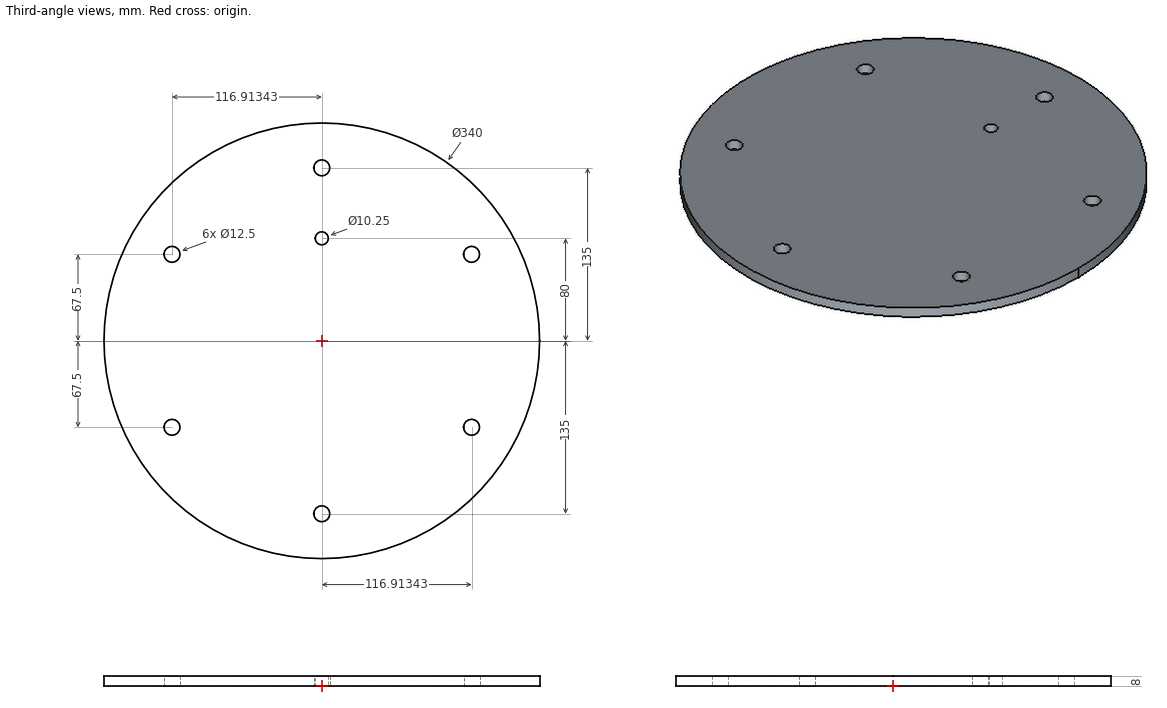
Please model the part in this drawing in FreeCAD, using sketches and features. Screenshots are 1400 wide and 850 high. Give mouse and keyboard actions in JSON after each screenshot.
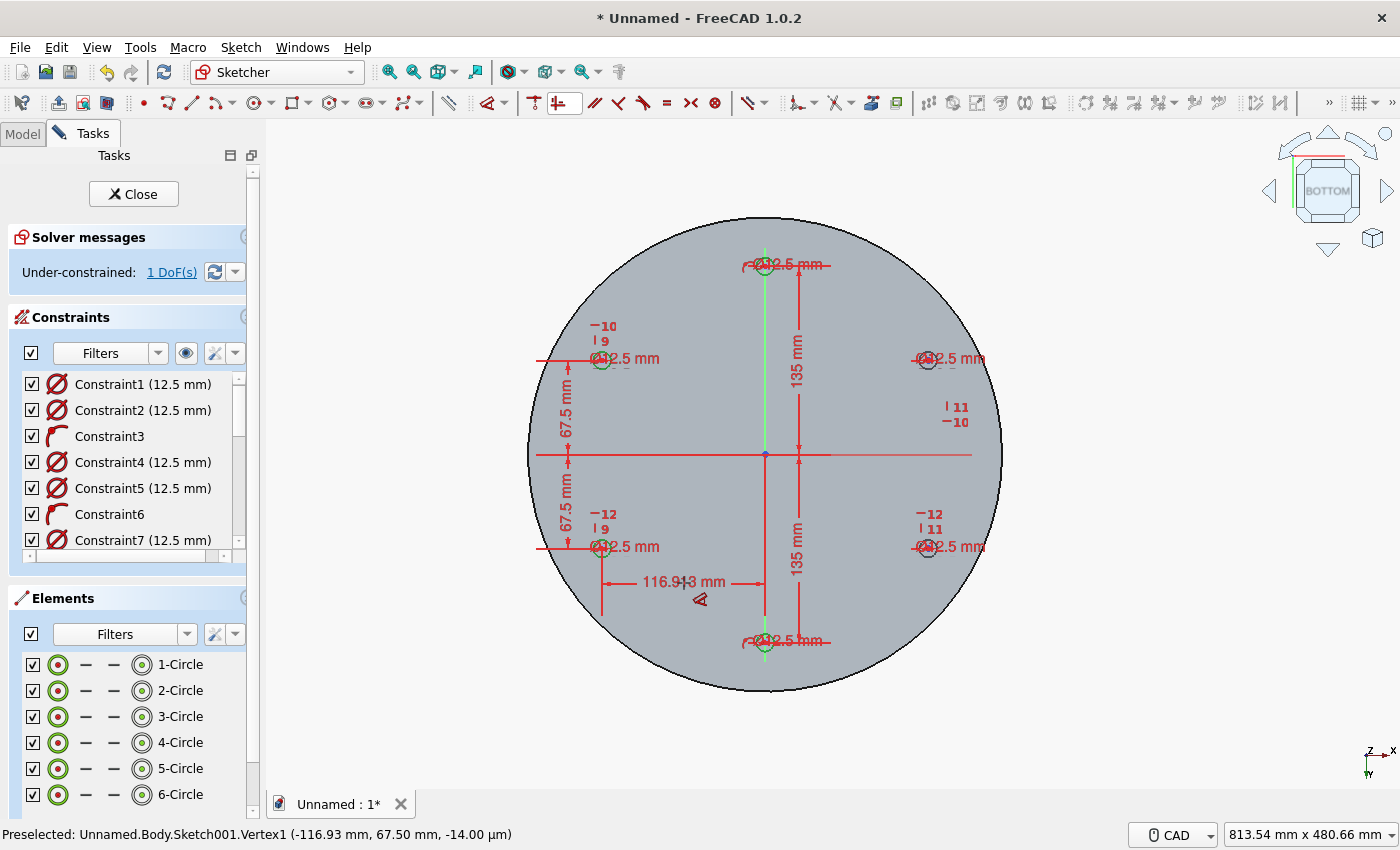
{"action": "left_click", "coordinate": [928, 361]}
{"action": "left_click", "coordinate": [847, 327]}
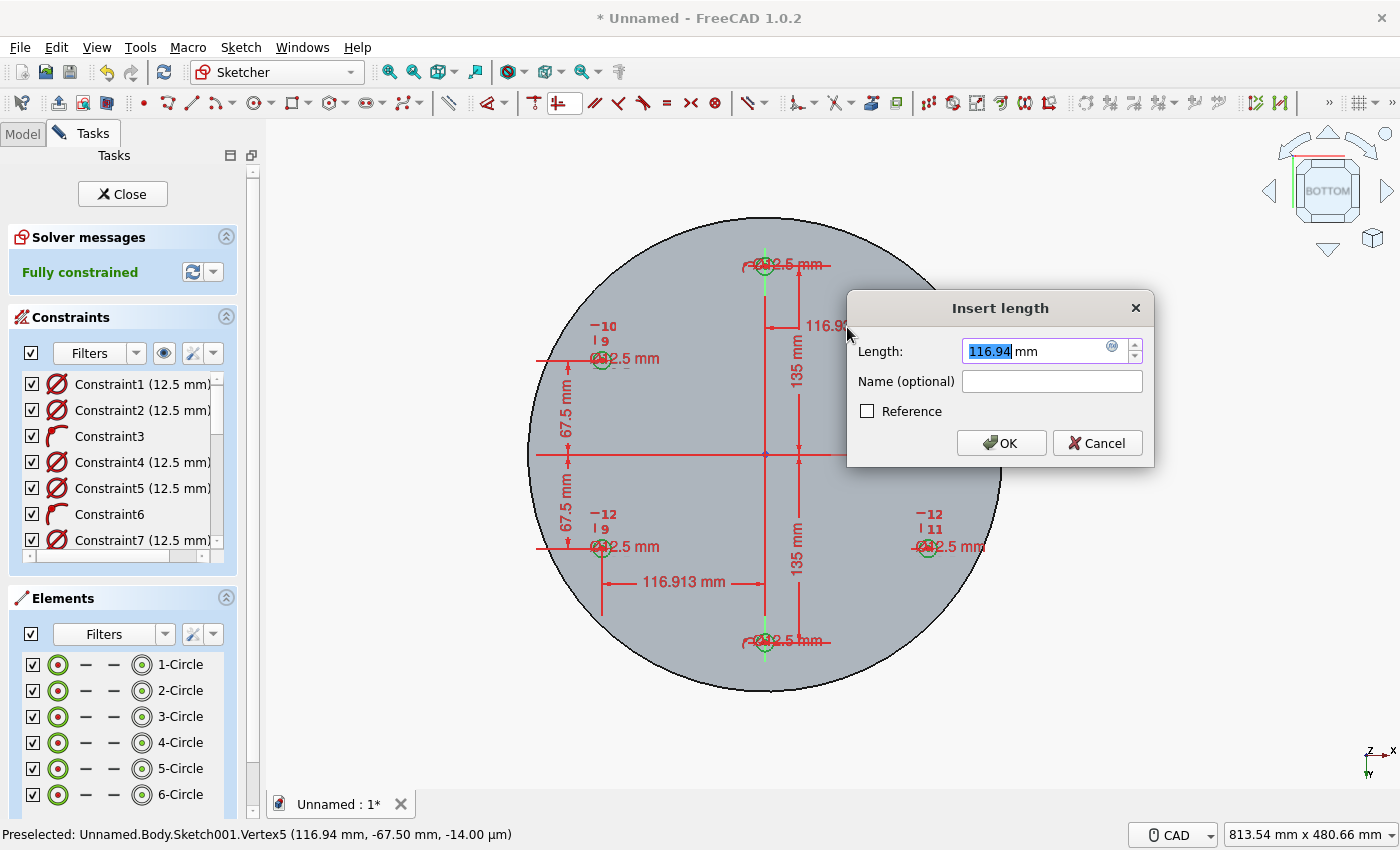
{"action": "type", "text": "116.91343"}
{"action": "key", "text": "Return"}
{"action": "key", "text": "Escape"}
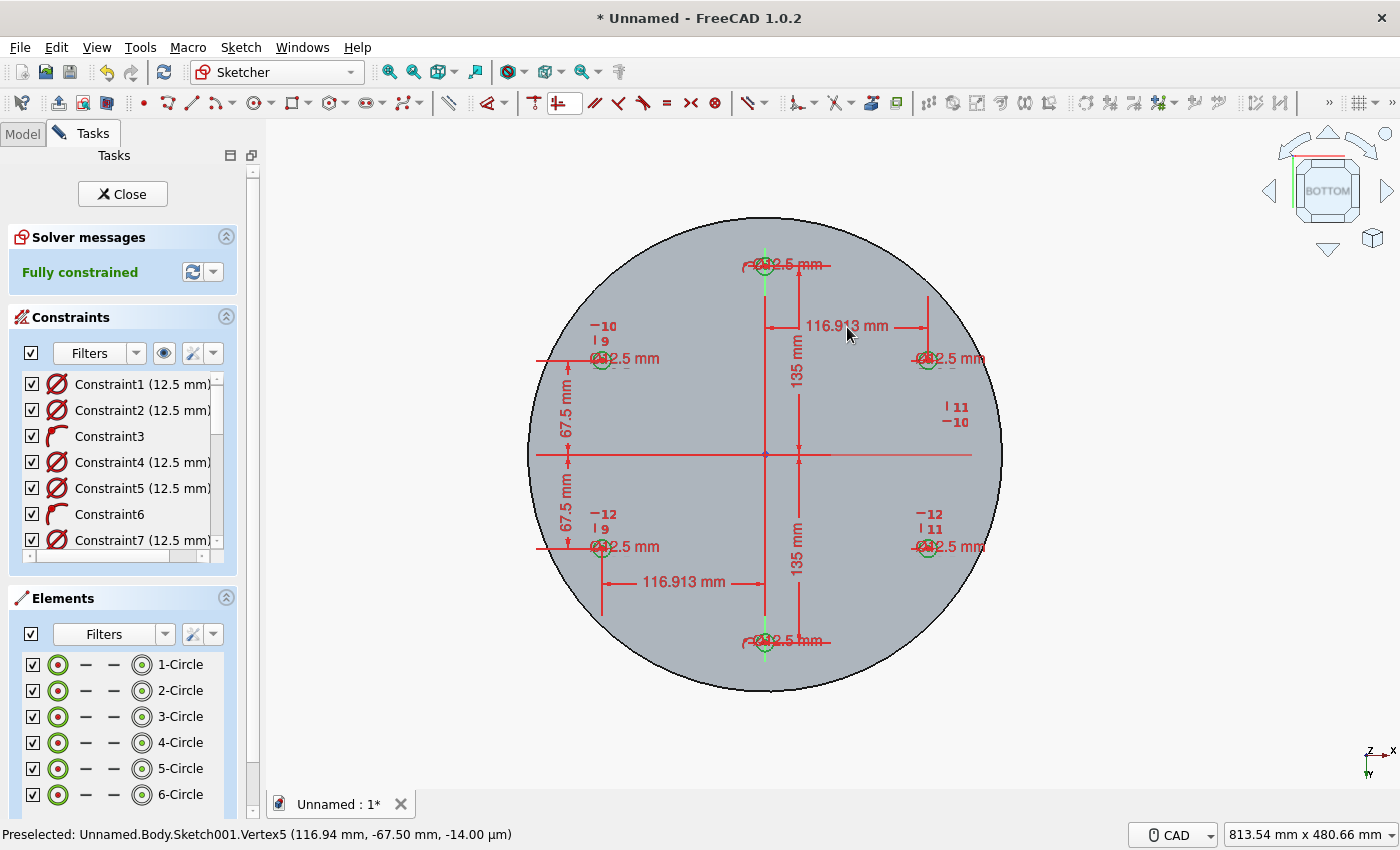
{"action": "left_click", "coordinate": [123, 194]}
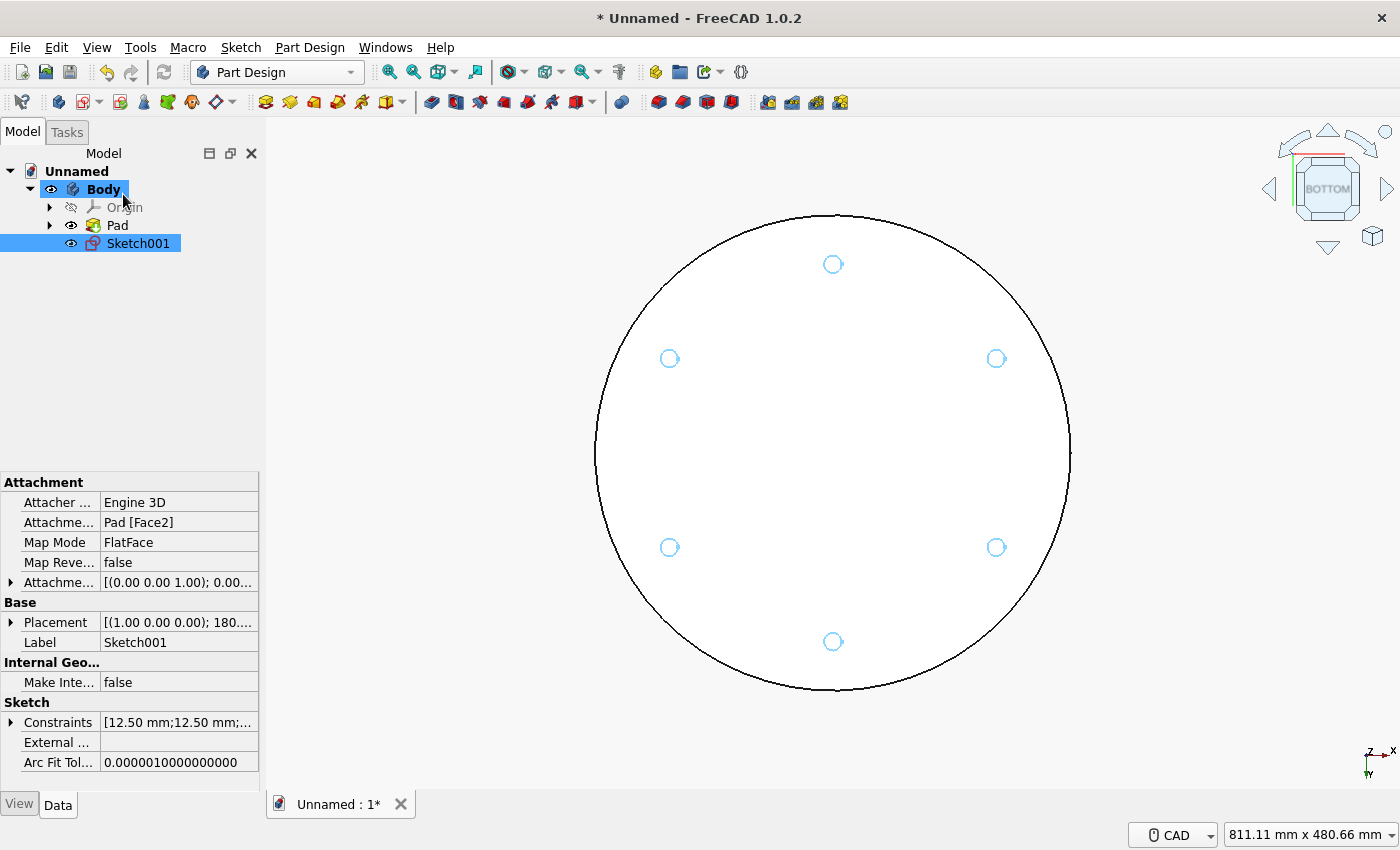
{"action": "left_click", "coordinate": [432, 102]}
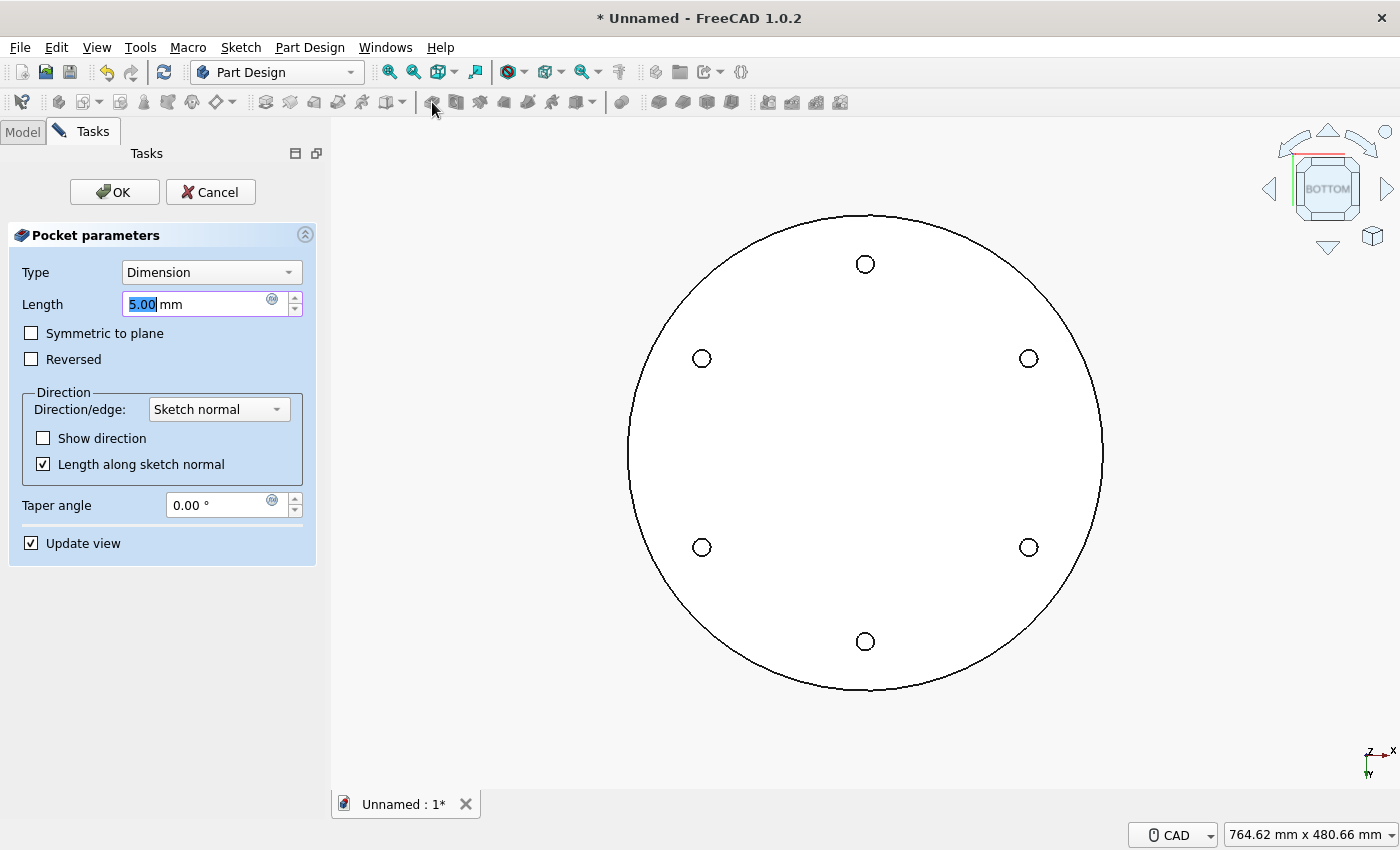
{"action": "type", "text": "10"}
{"action": "key", "text": "Tab"}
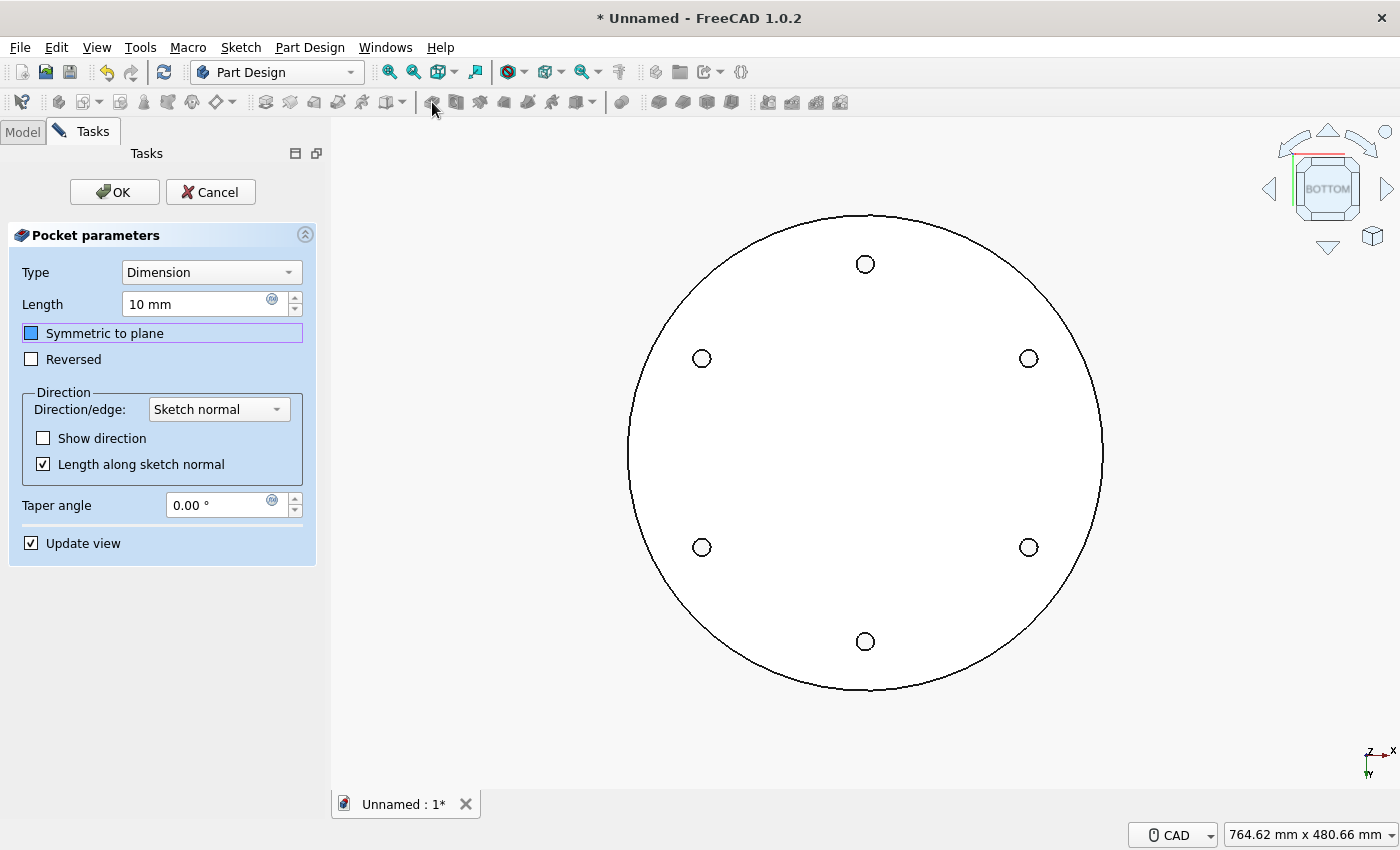
{"action": "left_click", "coordinate": [115, 192]}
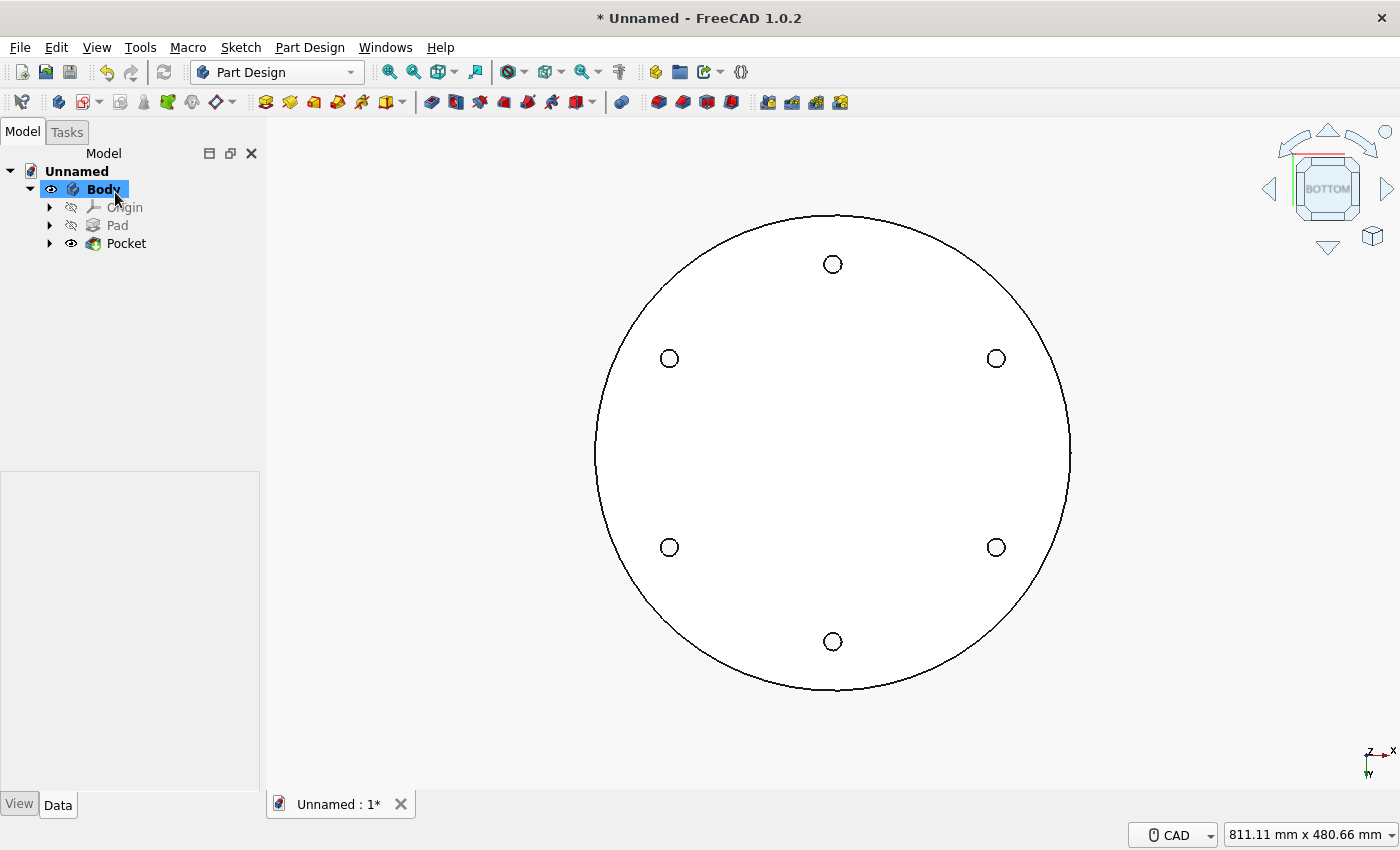
{"action": "left_click", "coordinate": [833, 452]}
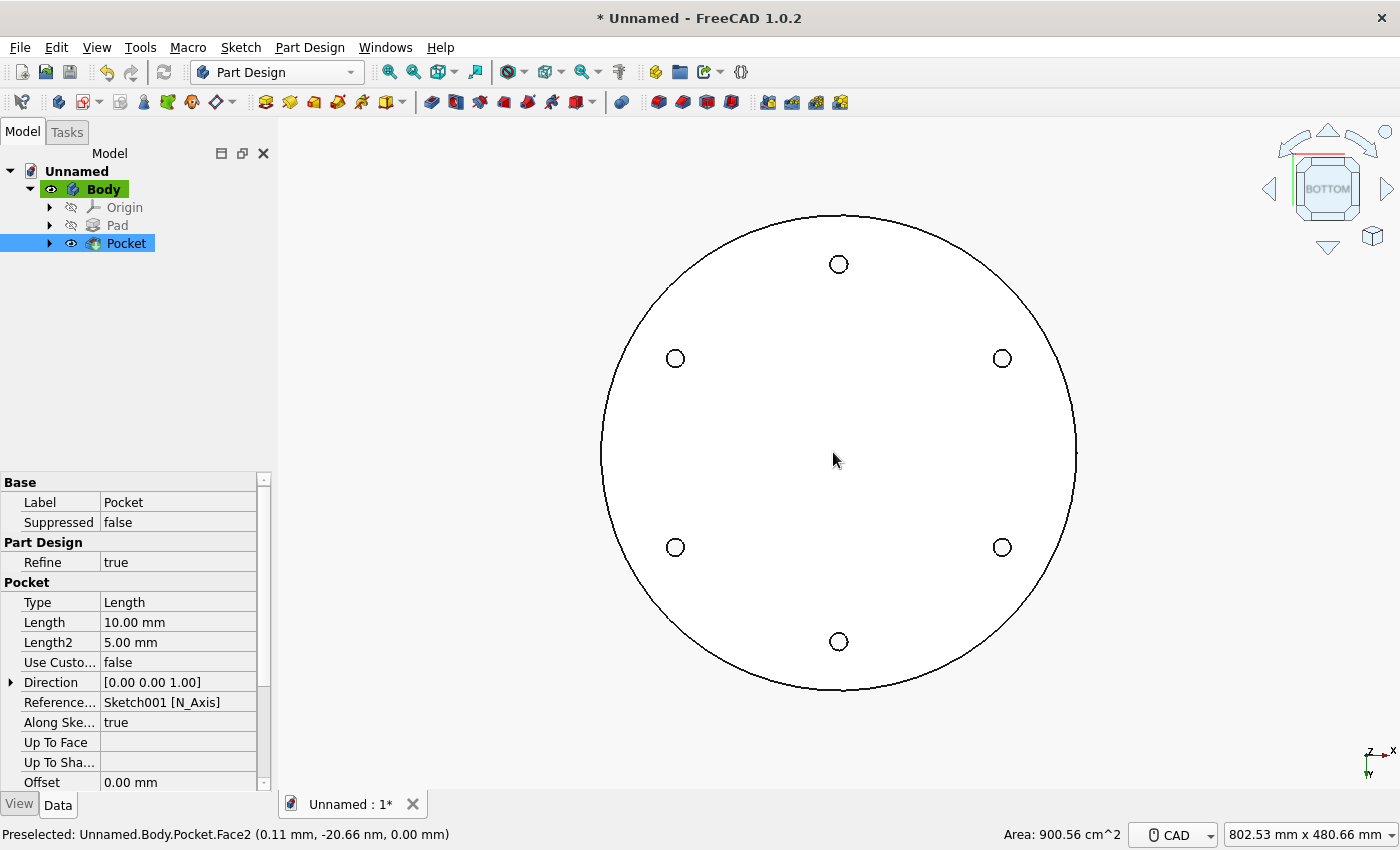
{"action": "left_click", "coordinate": [84, 102]}